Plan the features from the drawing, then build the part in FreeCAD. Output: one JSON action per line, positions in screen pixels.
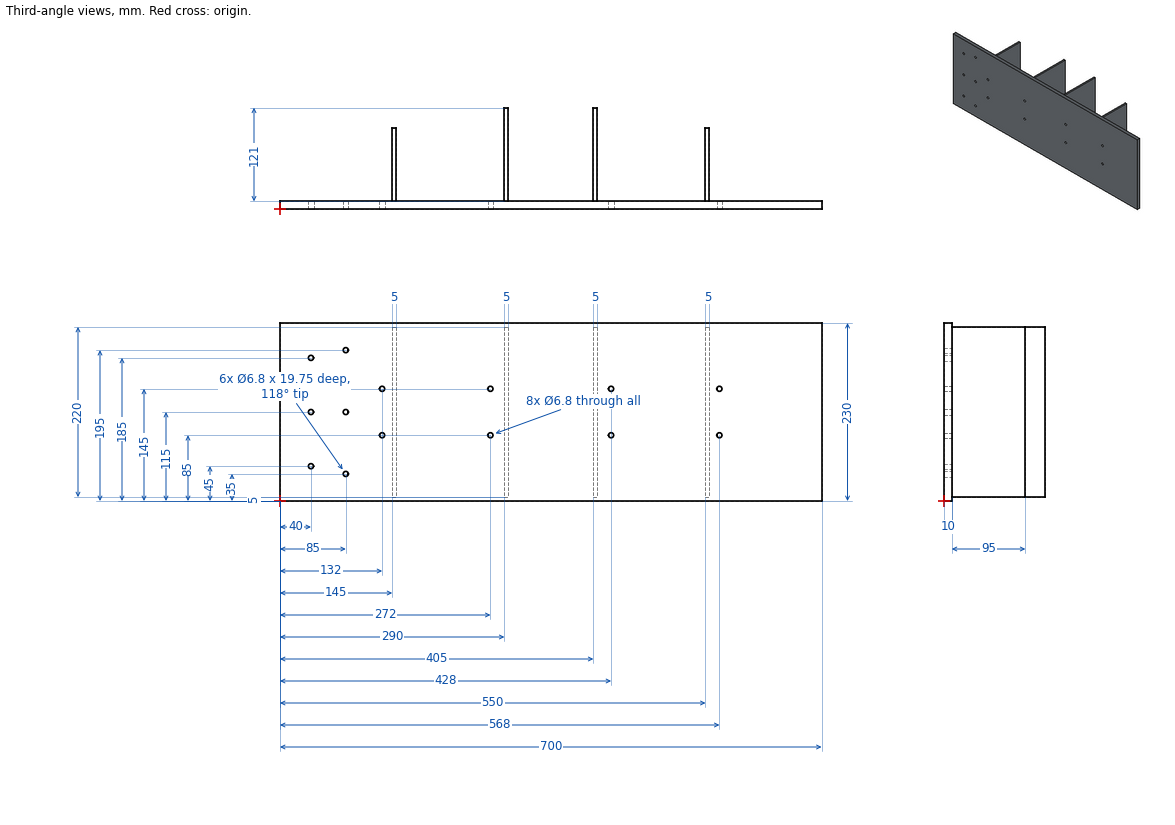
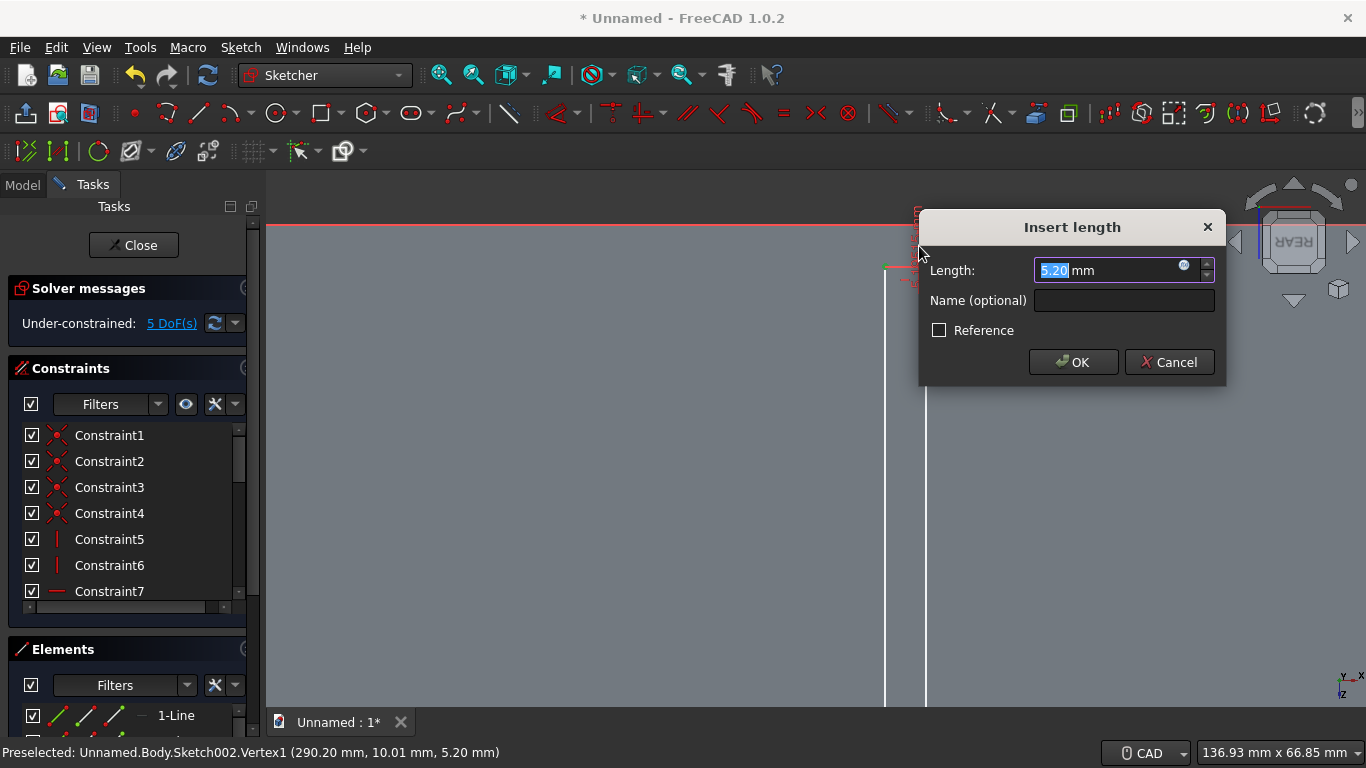
{"action": "type", "text": "5"}
{"action": "key", "text": "Return"}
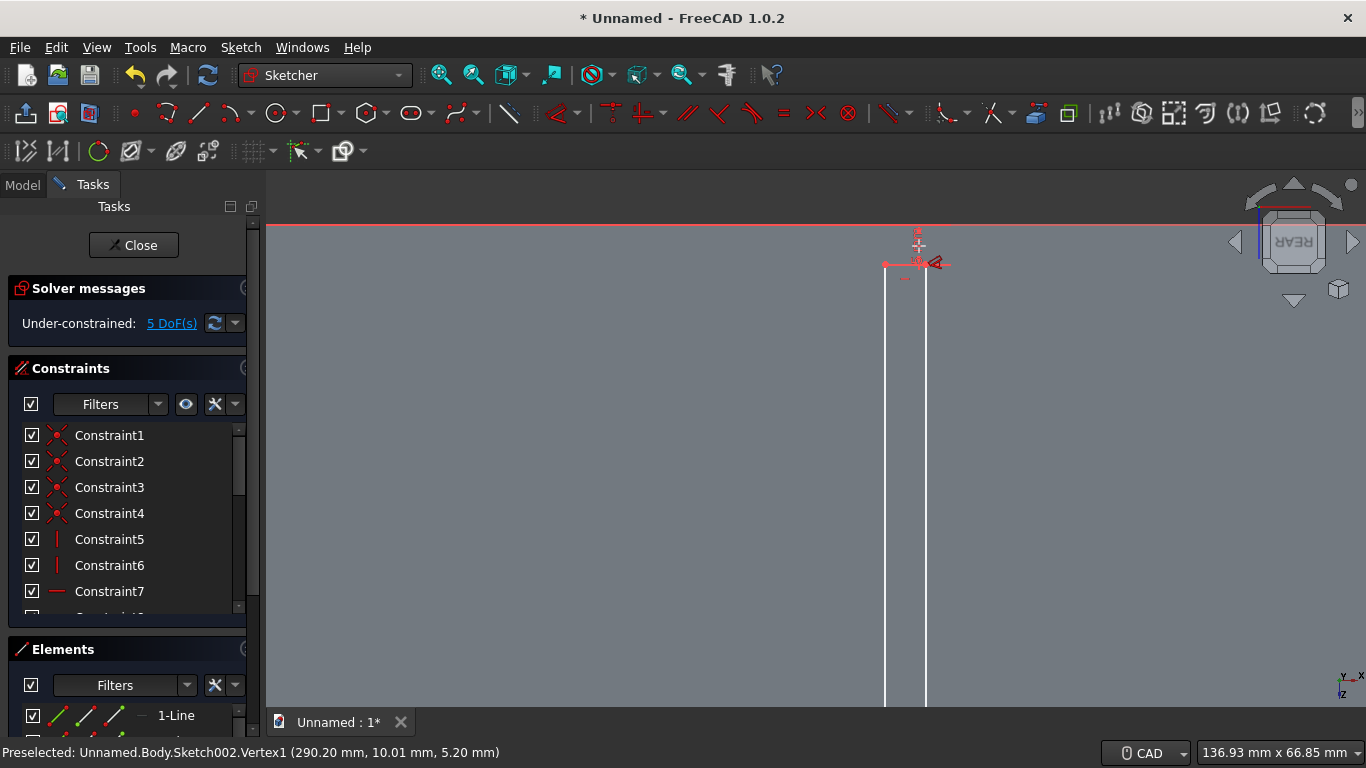
{"action": "scroll", "coordinate": [886, 264], "scroll_direction": "down", "scroll_amount": 8}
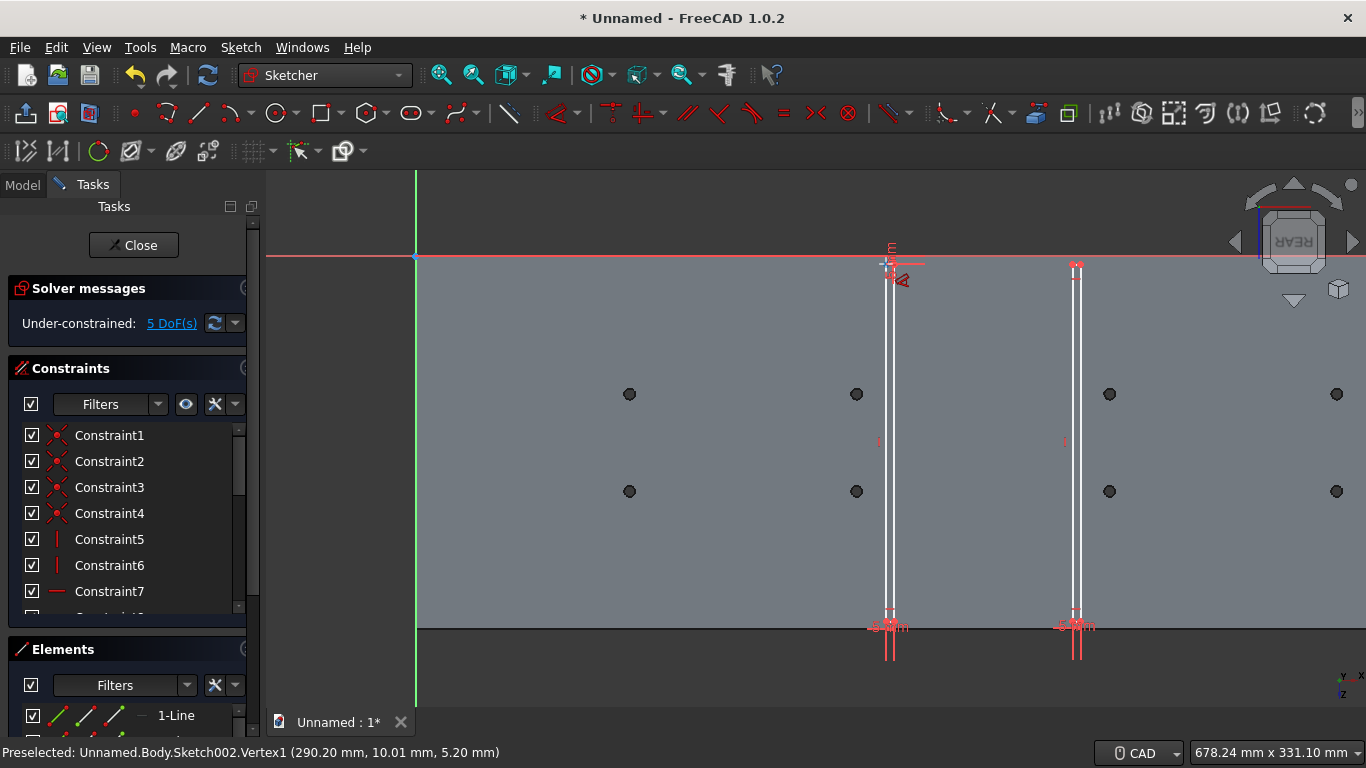
{"action": "scroll", "coordinate": [1073, 265], "scroll_direction": "up", "scroll_amount": 8}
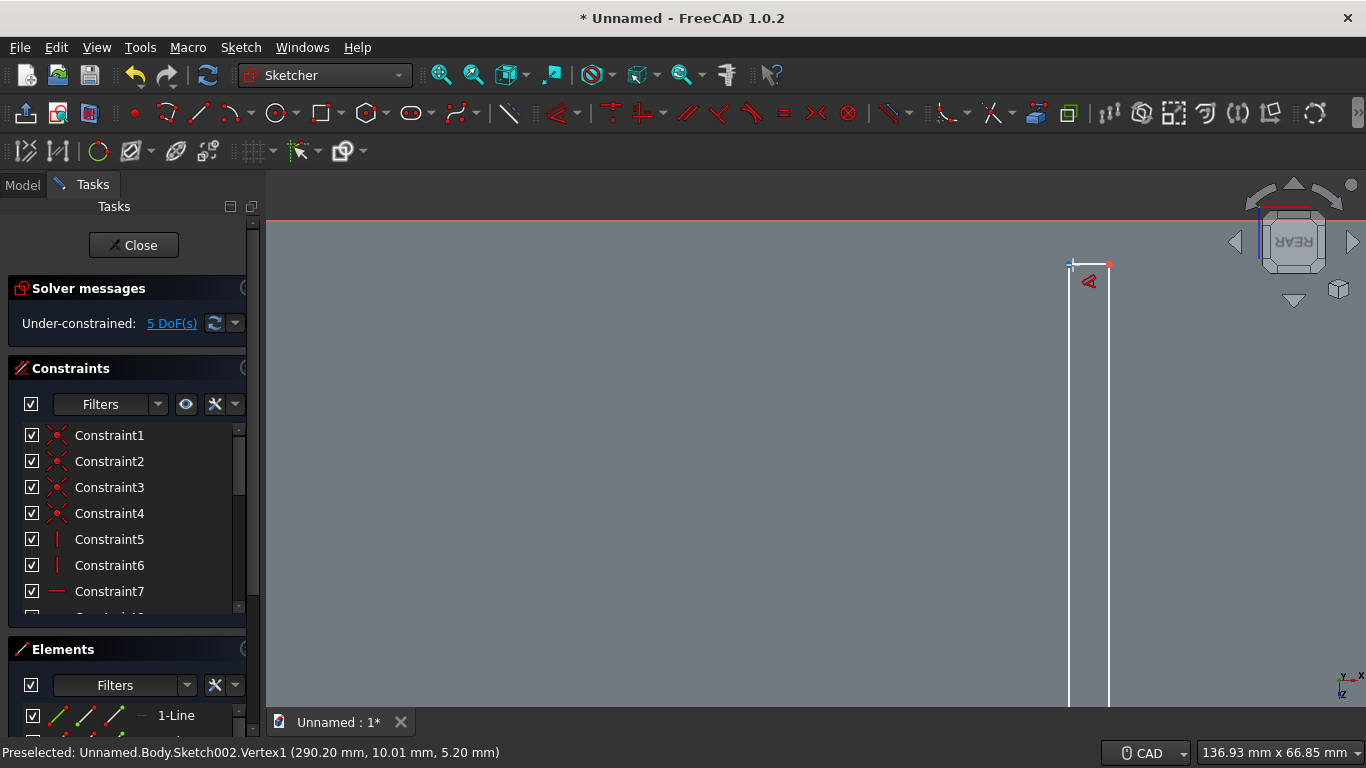
{"action": "left_click", "coordinate": [1069, 264]}
{"action": "left_click", "coordinate": [1103, 243]}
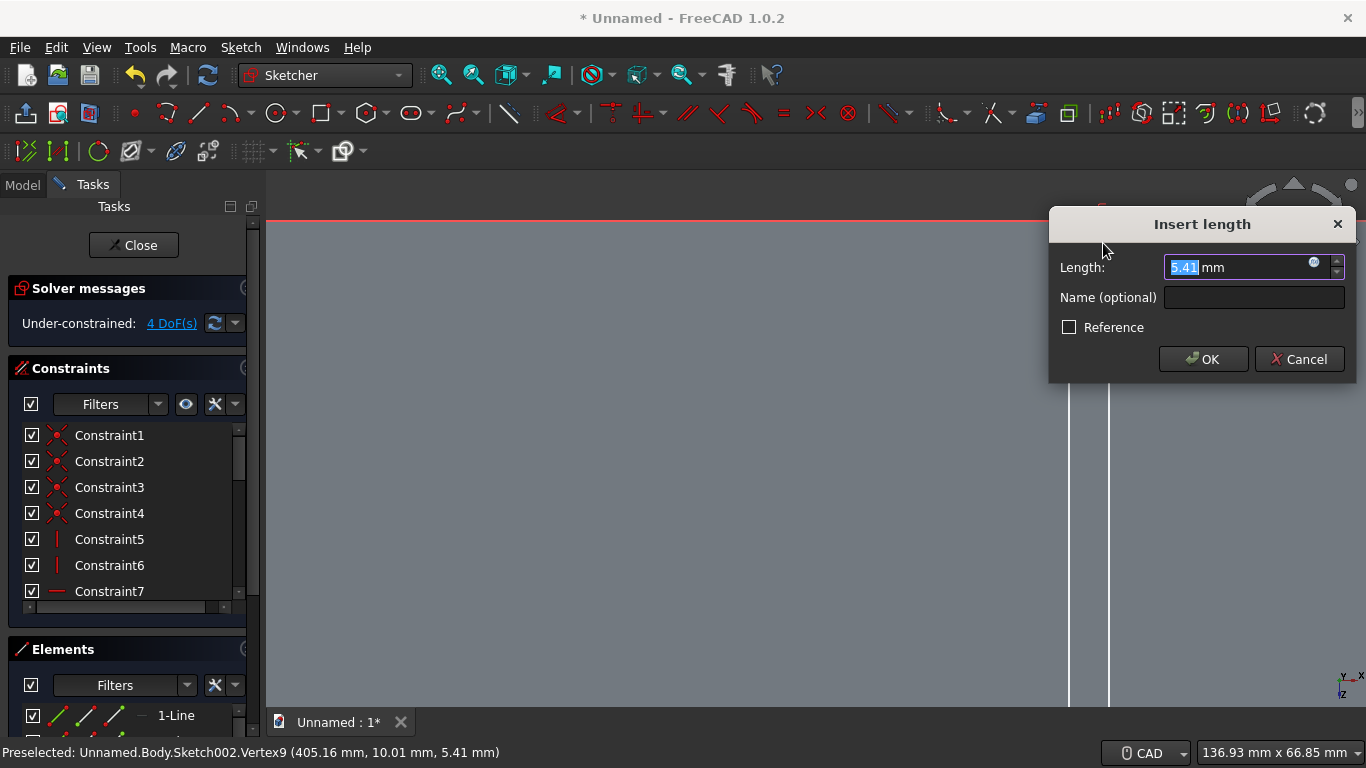
{"action": "type", "text": "5"}
{"action": "key", "text": "Return"}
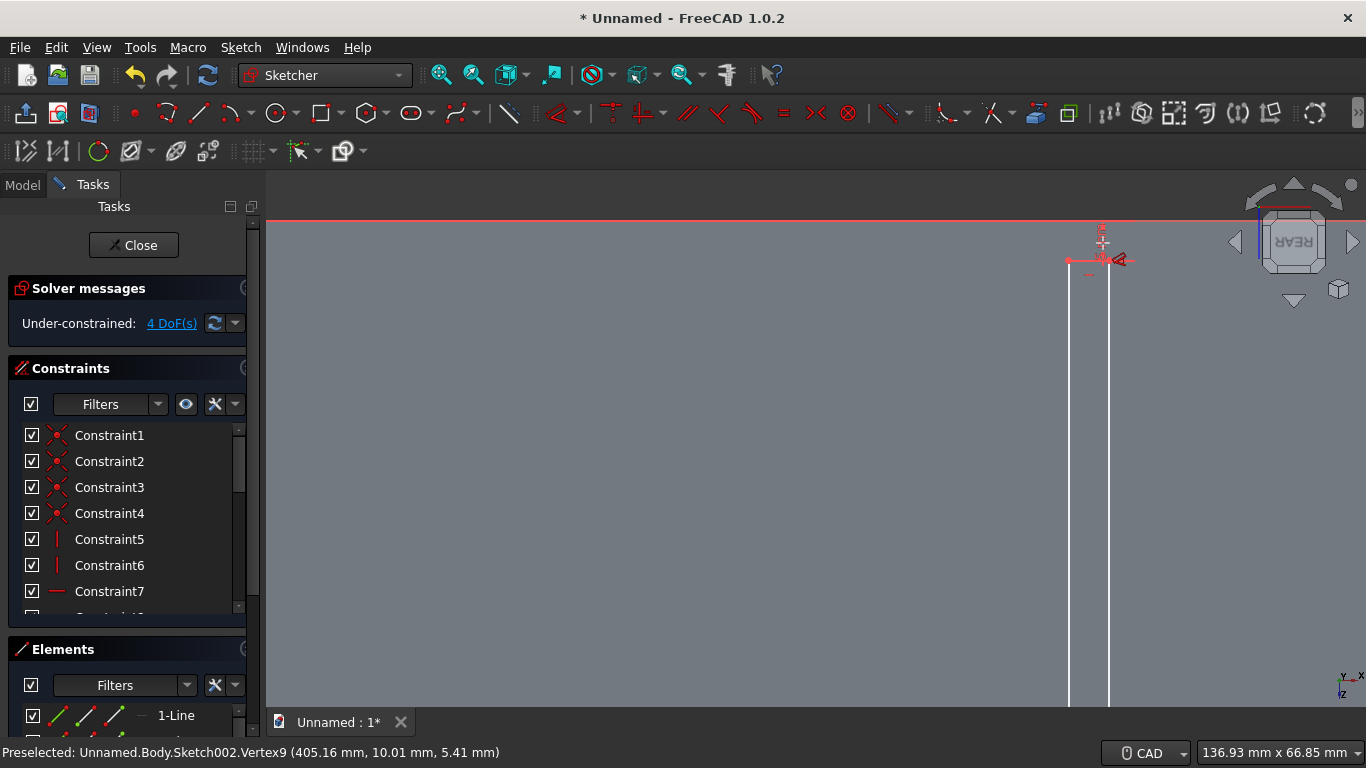
{"action": "scroll", "coordinate": [1073, 265], "scroll_direction": "down", "scroll_amount": 8}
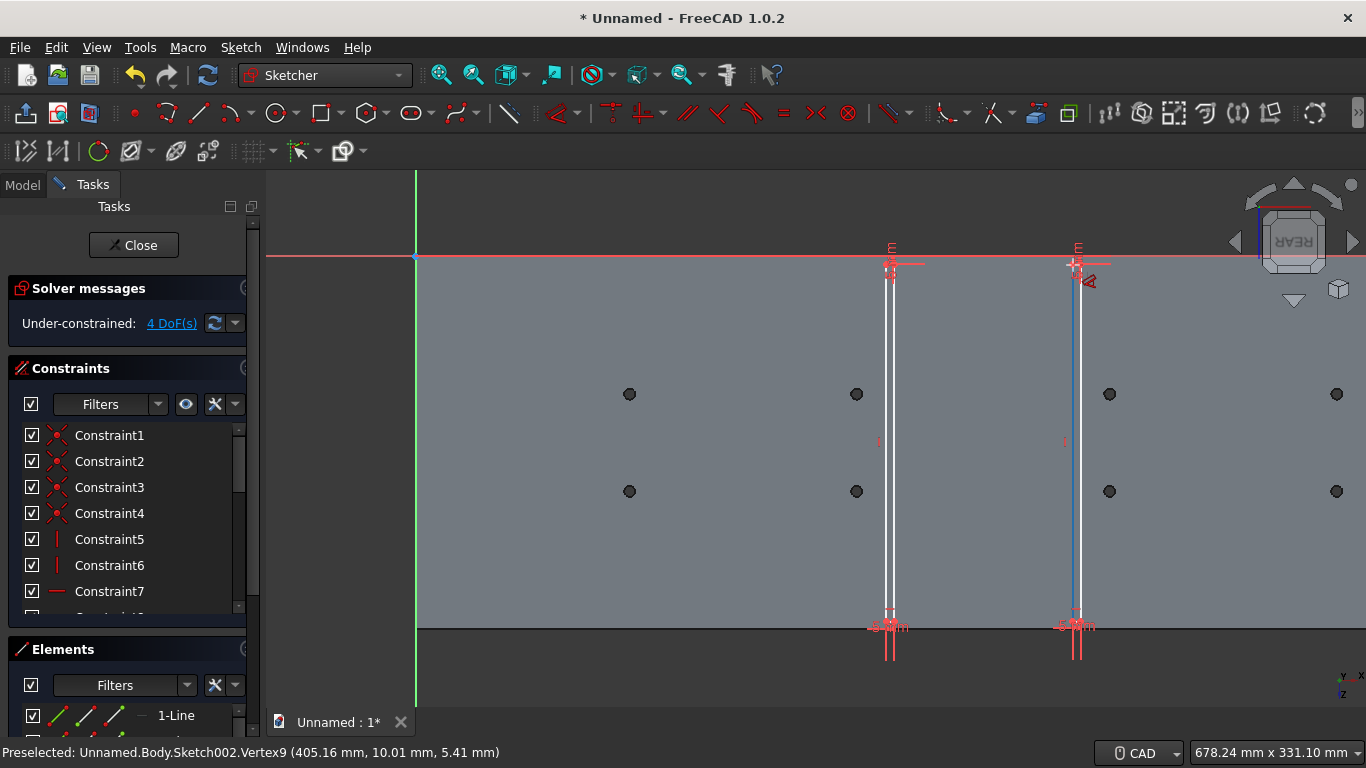
{"action": "scroll", "coordinate": [886, 372], "scroll_direction": "up", "scroll_amount": 3}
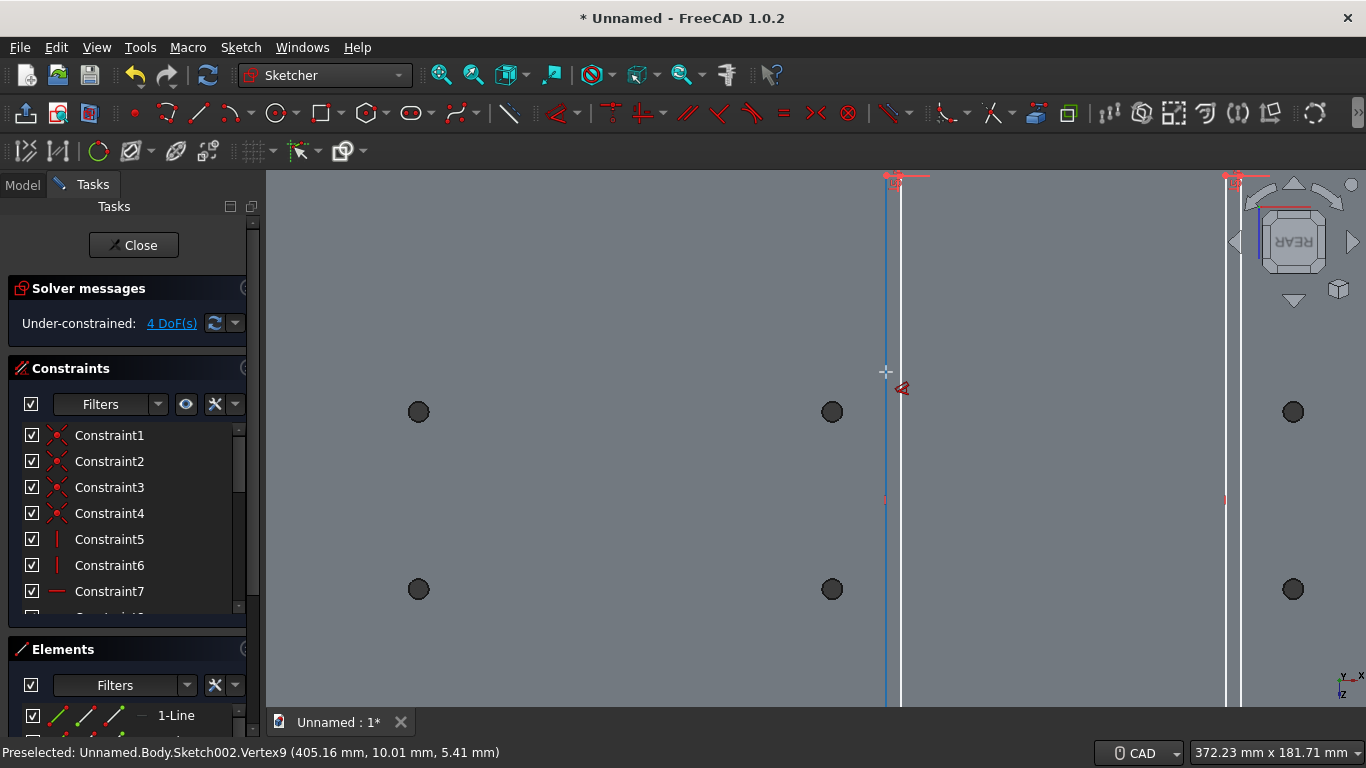
{"action": "left_click", "coordinate": [886, 371]}
{"action": "left_click", "coordinate": [920, 438]}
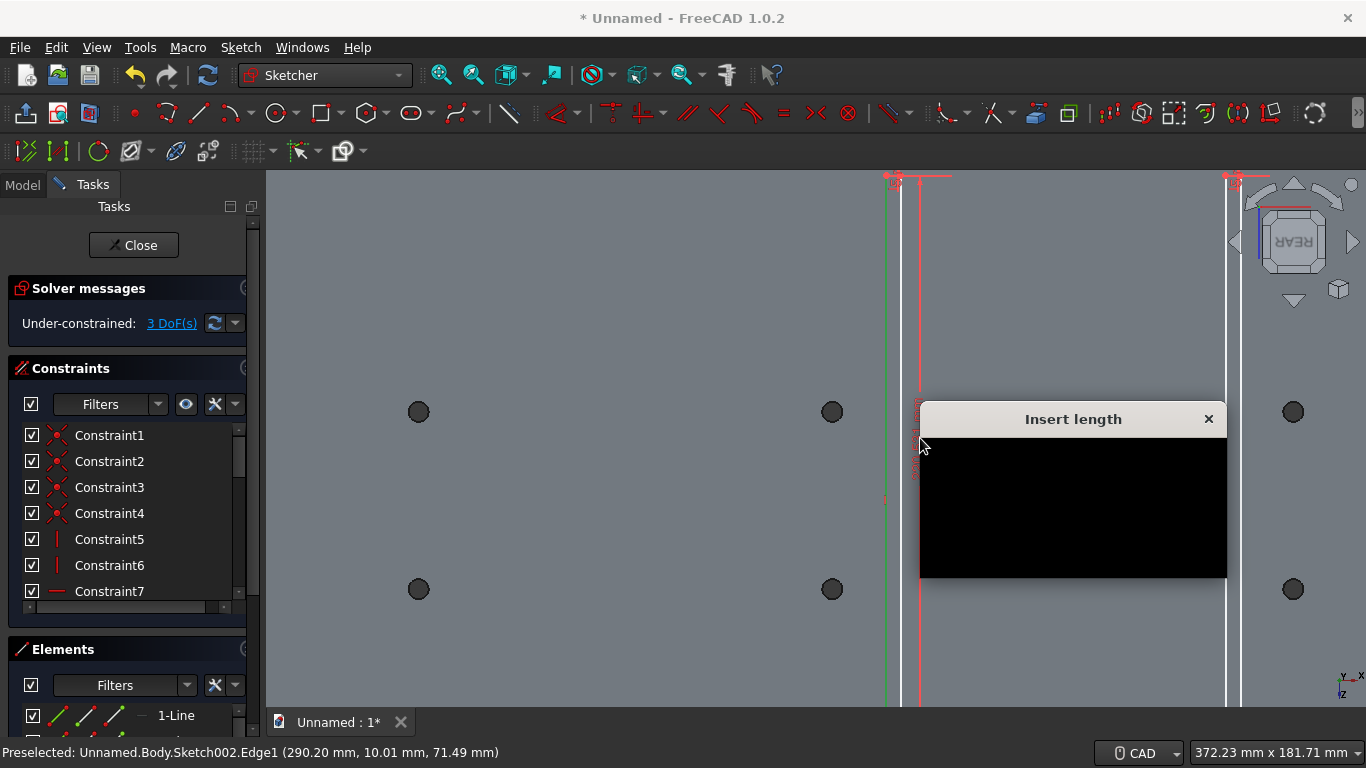
{"action": "type", "text": "220"}
{"action": "key", "text": "Return"}